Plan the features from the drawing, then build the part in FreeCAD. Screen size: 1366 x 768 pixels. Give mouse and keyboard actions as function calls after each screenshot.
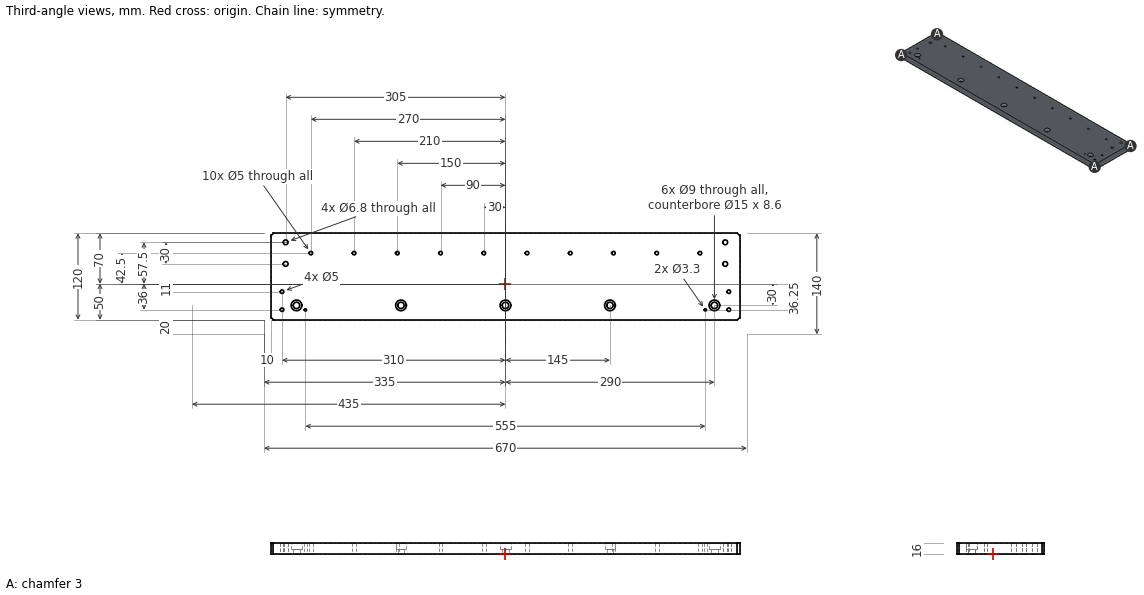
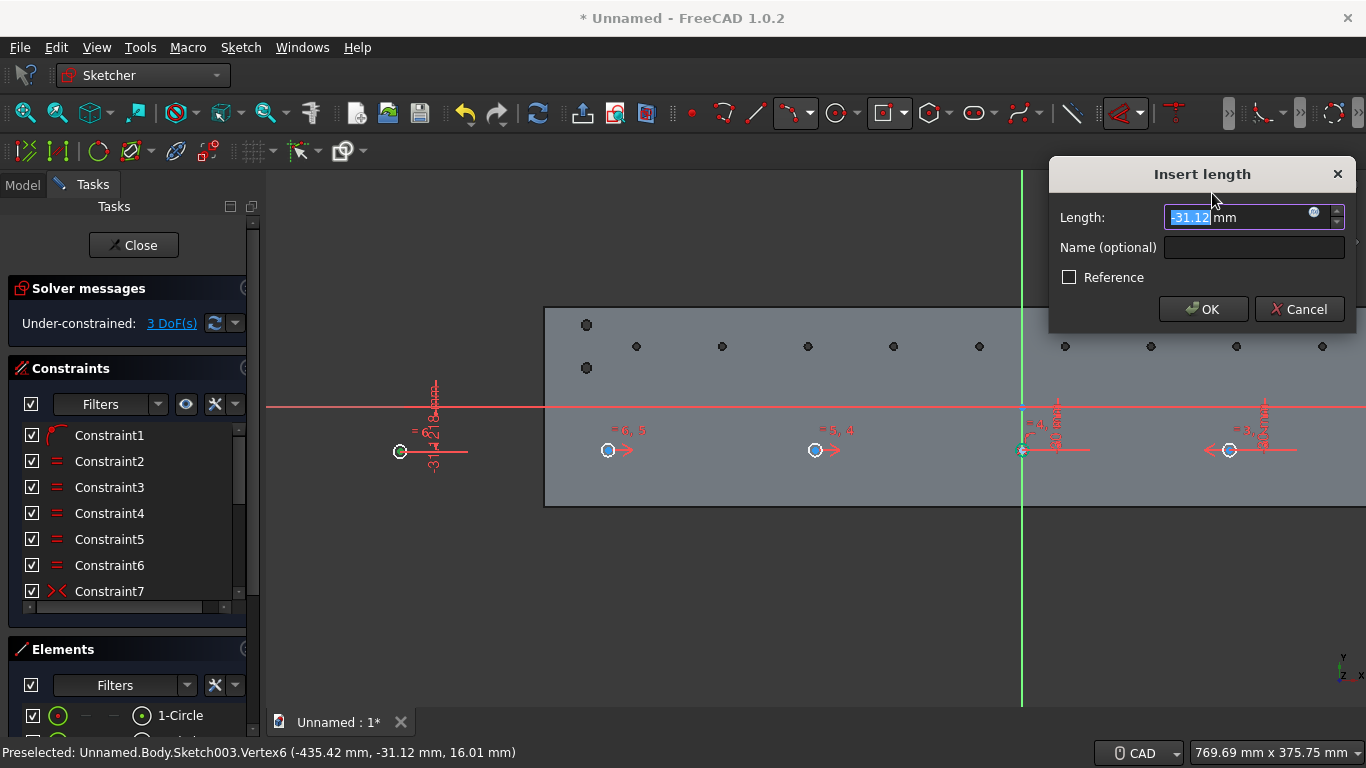
text(-30)
key(Return)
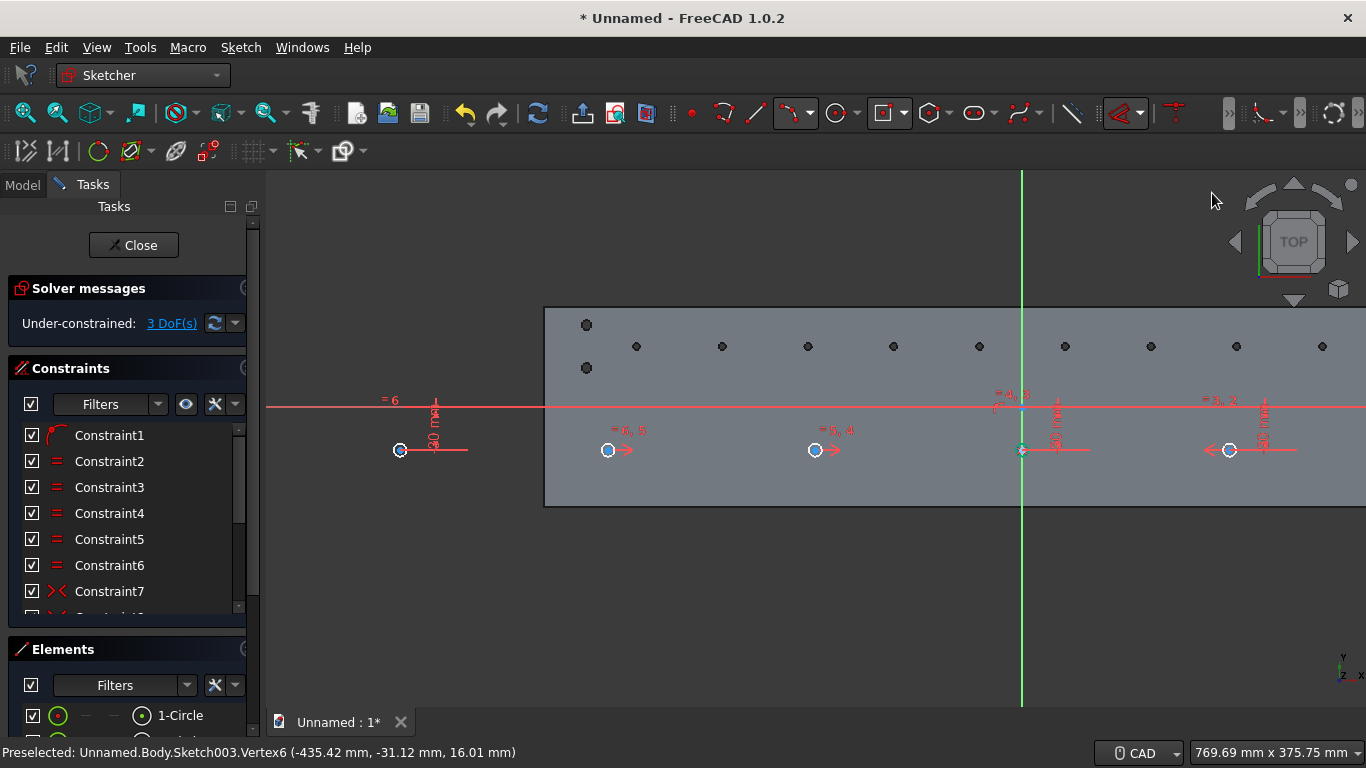
scroll(399, 452, down, 2)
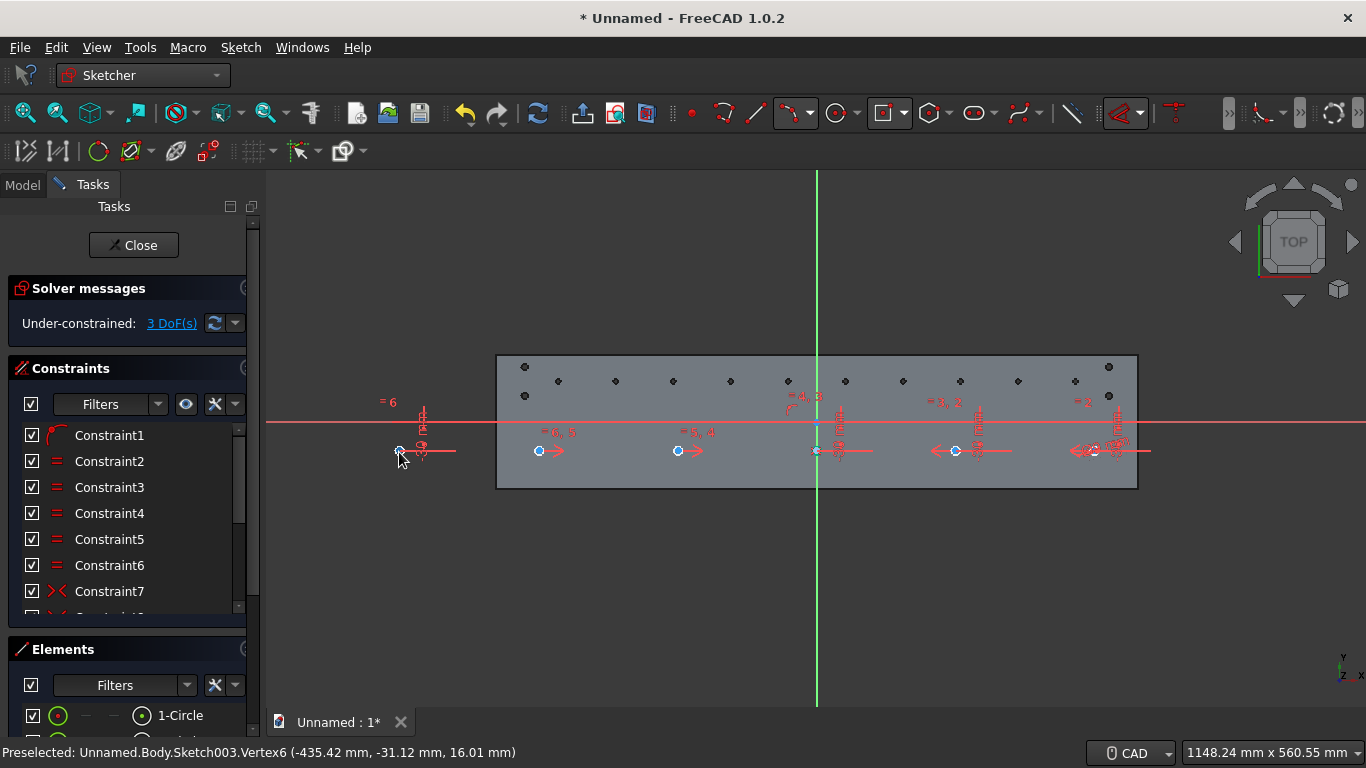
click(1095, 451)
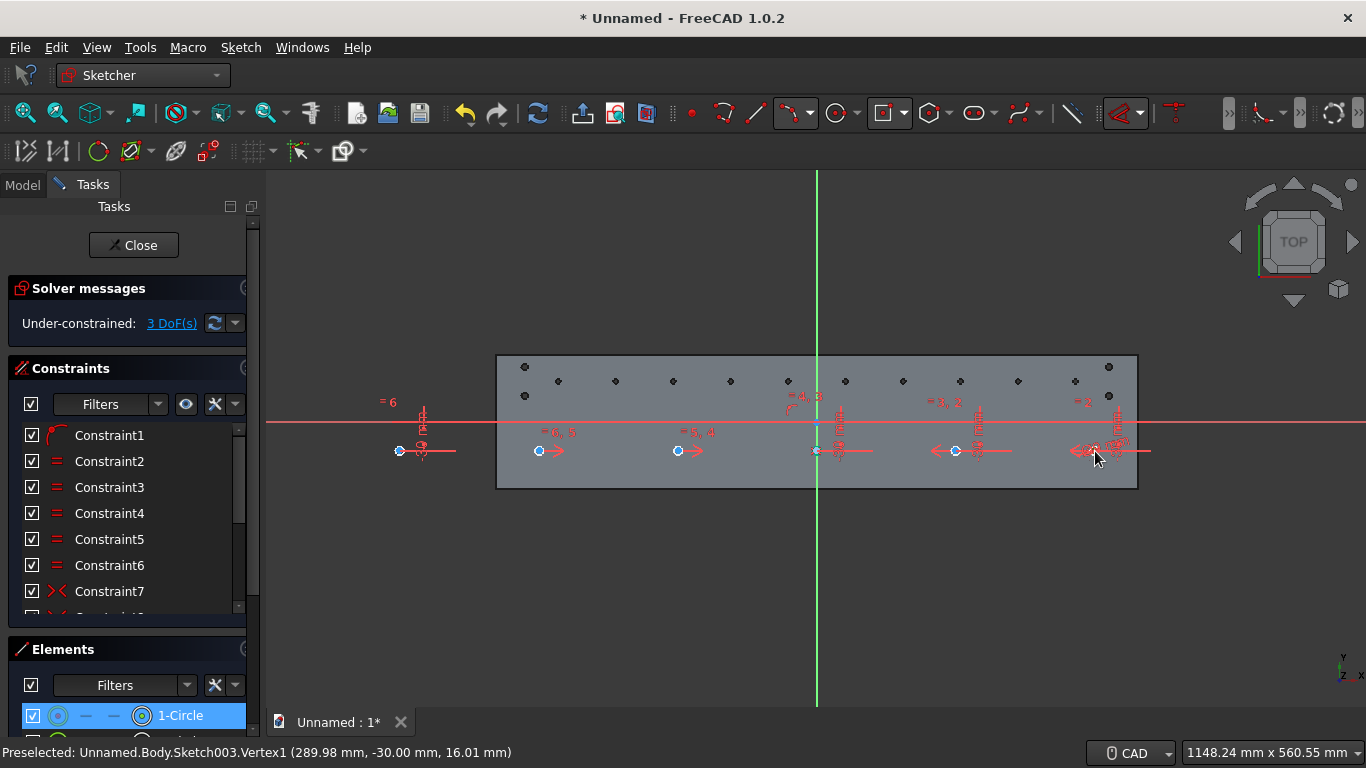
click(1142, 114)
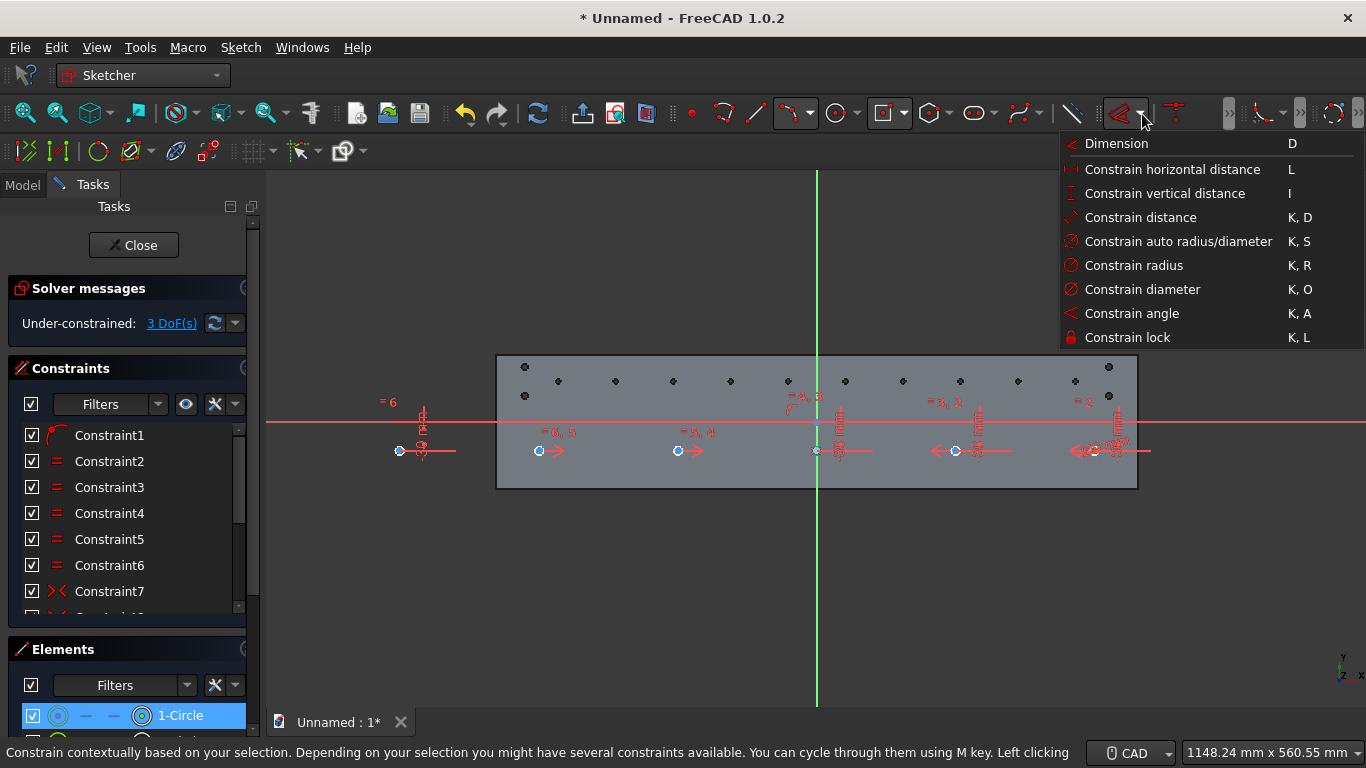
click(1212, 169)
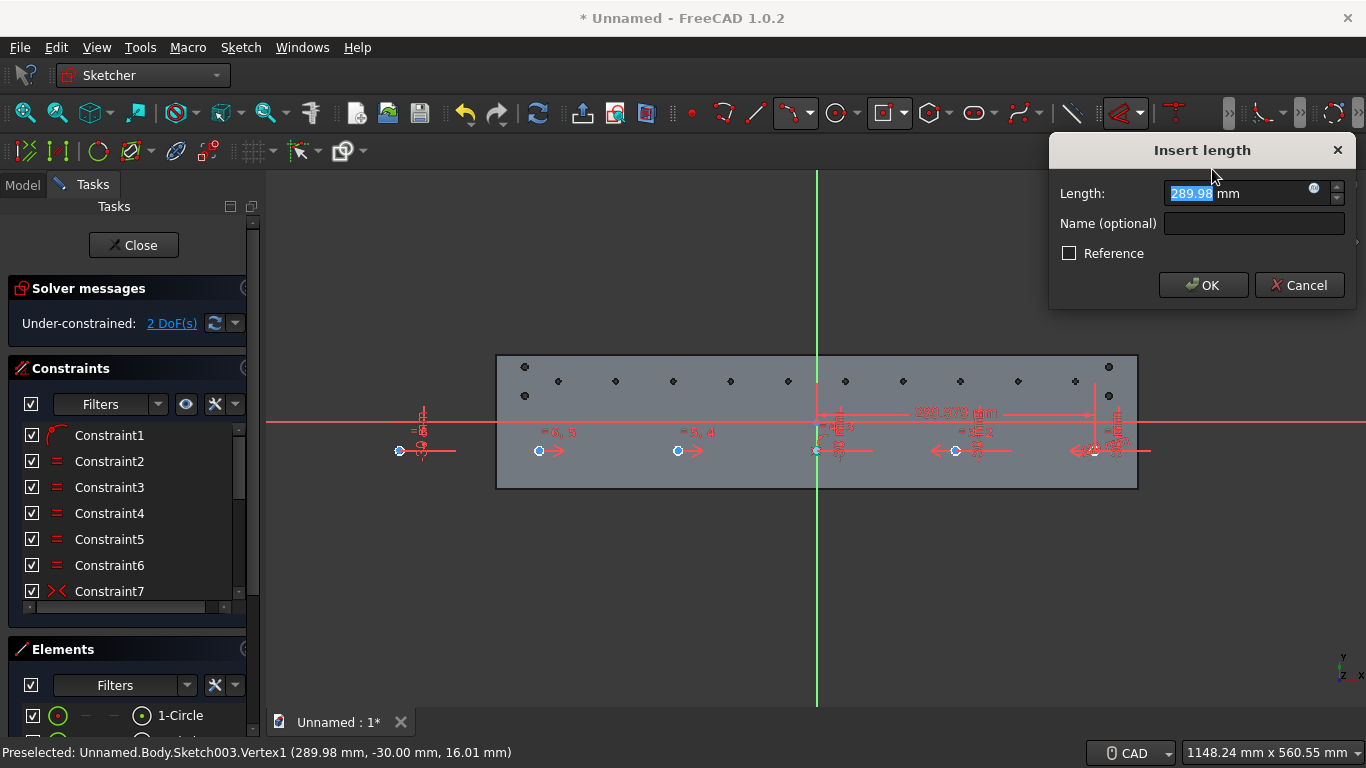
text(290)
key(Return)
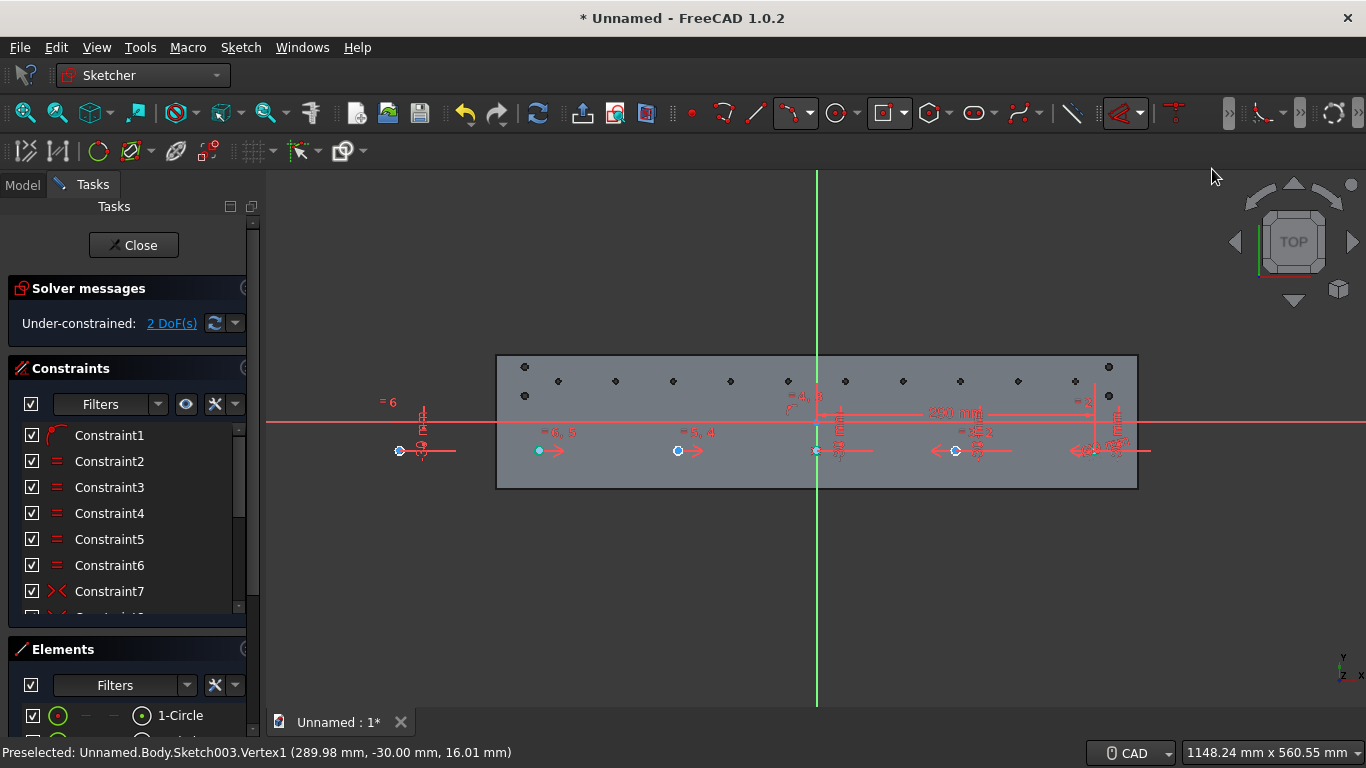
click(956, 451)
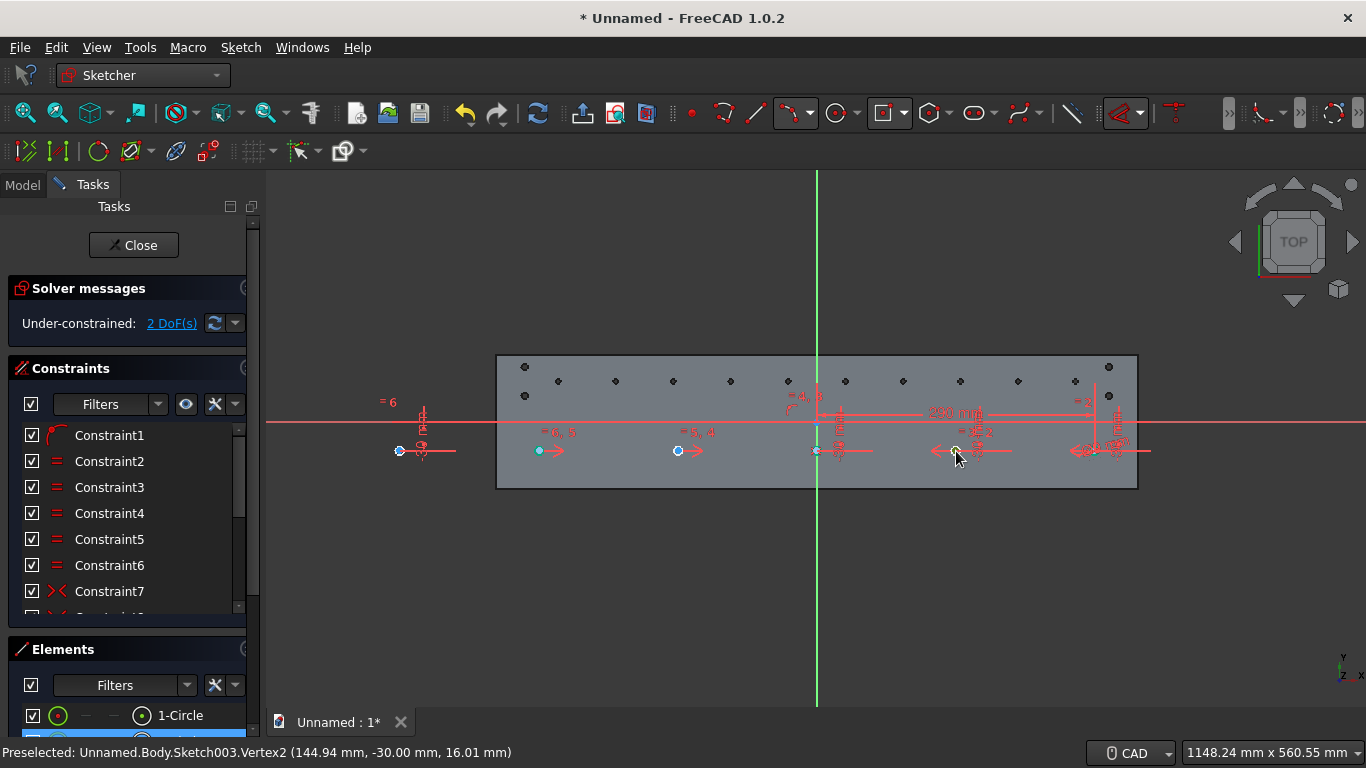
click(1142, 114)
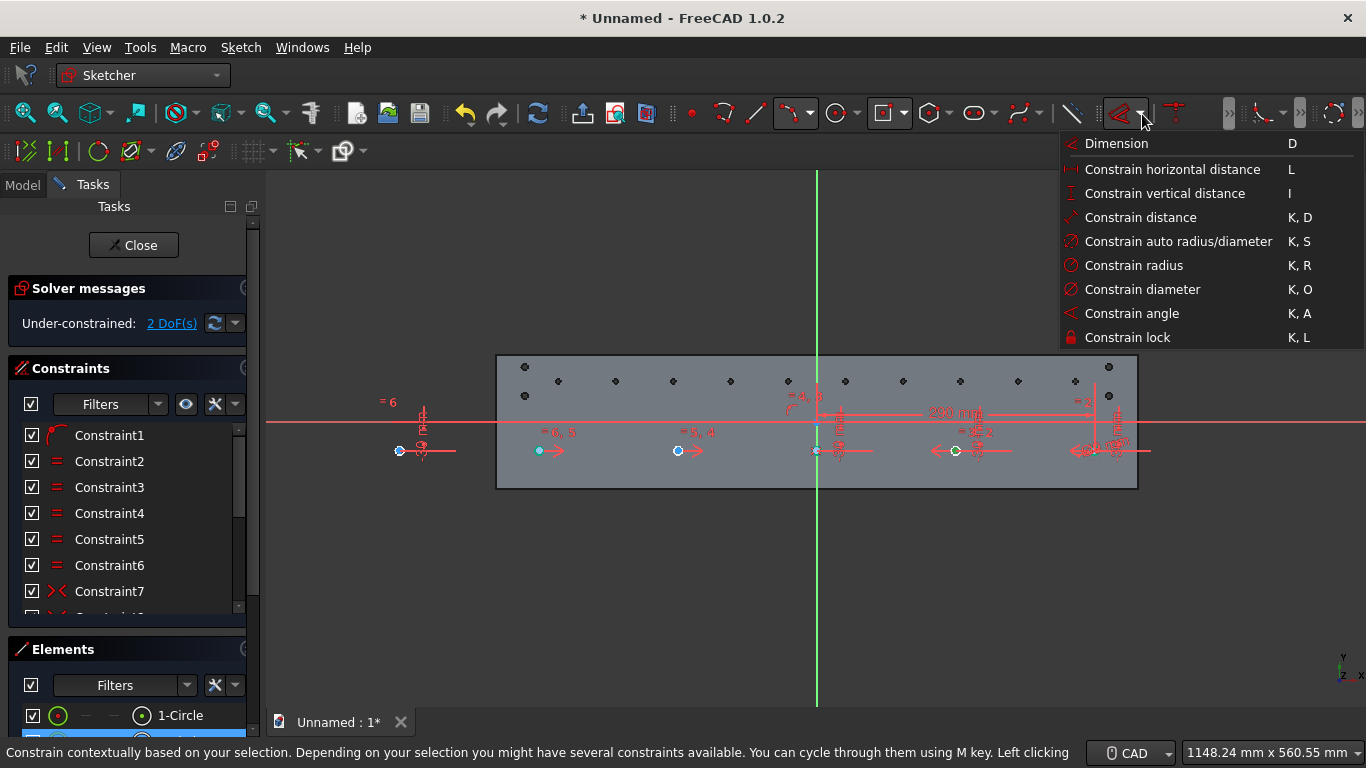
click(1212, 169)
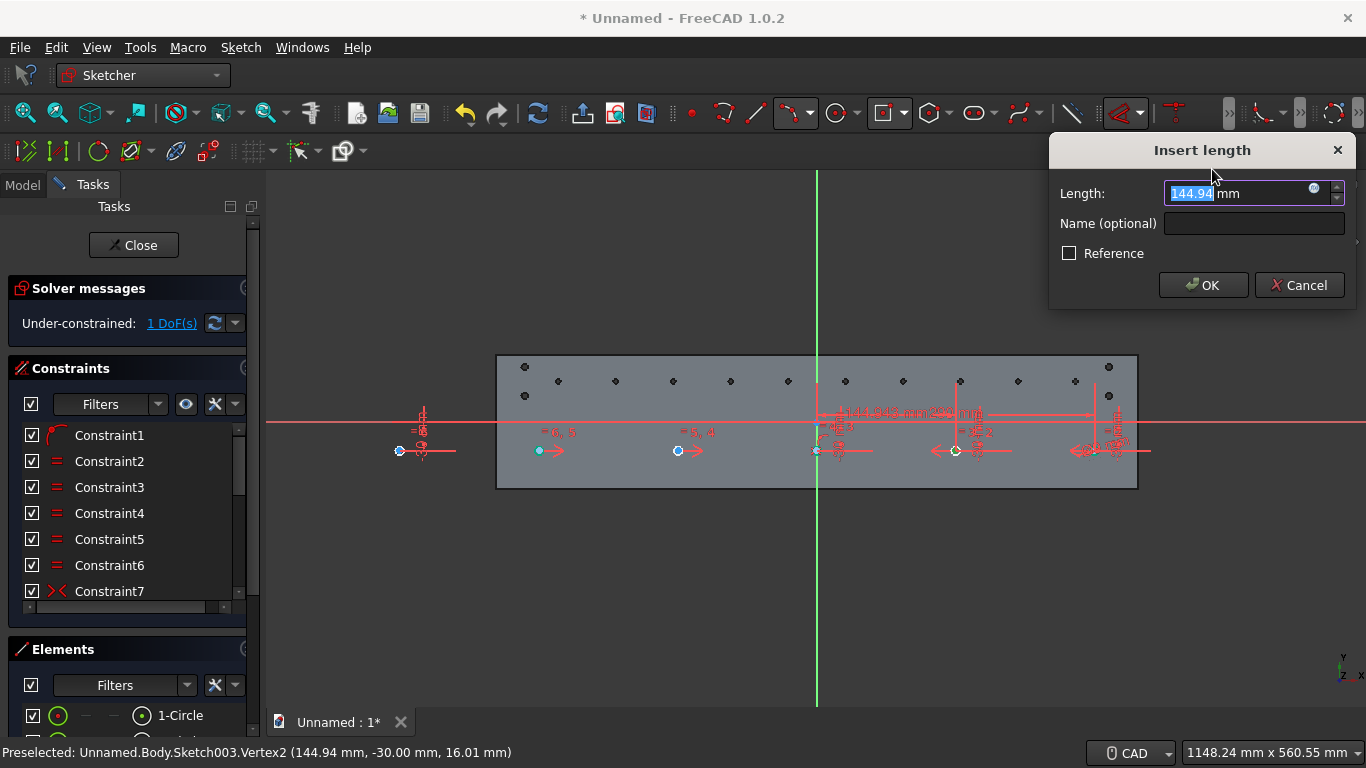
text(145)
key(Return)